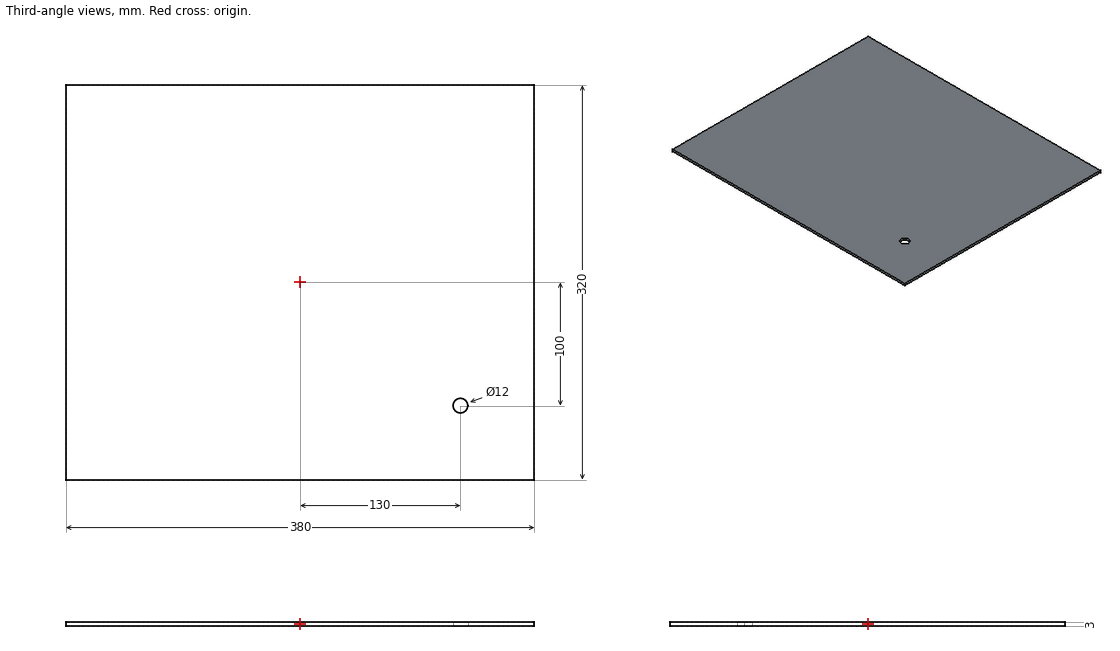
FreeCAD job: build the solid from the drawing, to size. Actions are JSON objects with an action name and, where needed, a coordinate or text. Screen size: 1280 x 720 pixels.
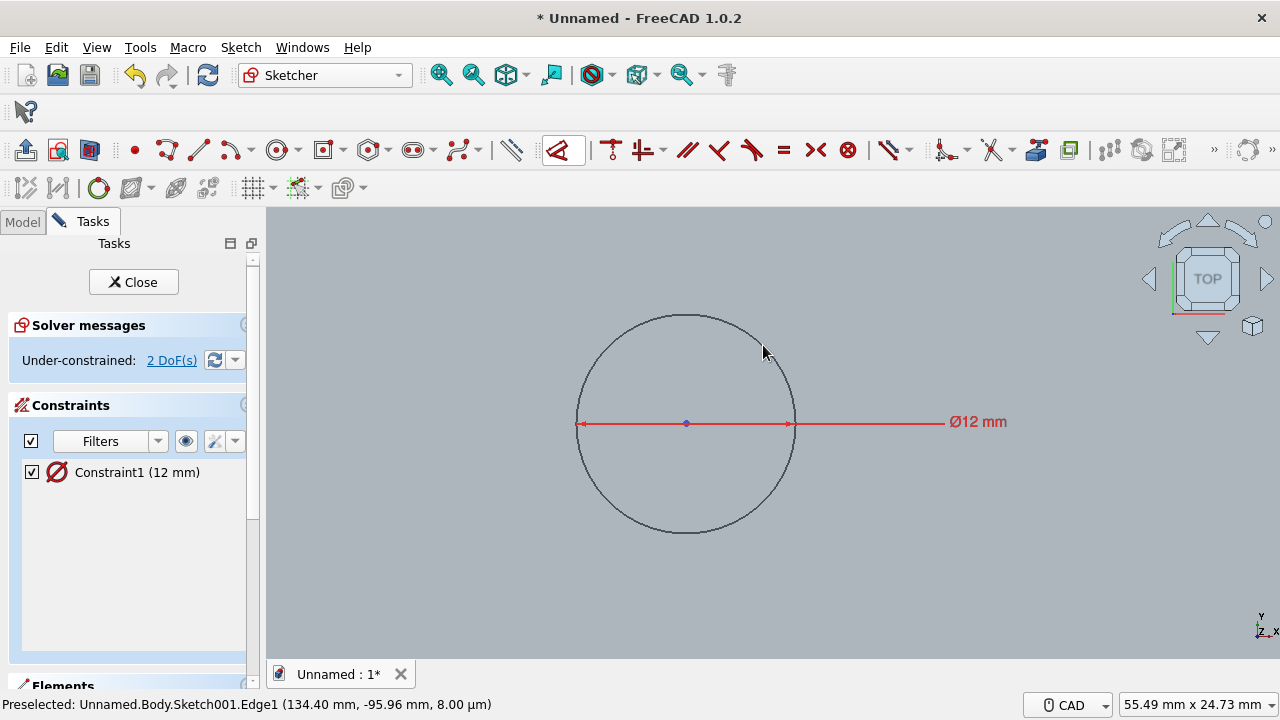
{"action": "left_click", "coordinate": [558, 150]}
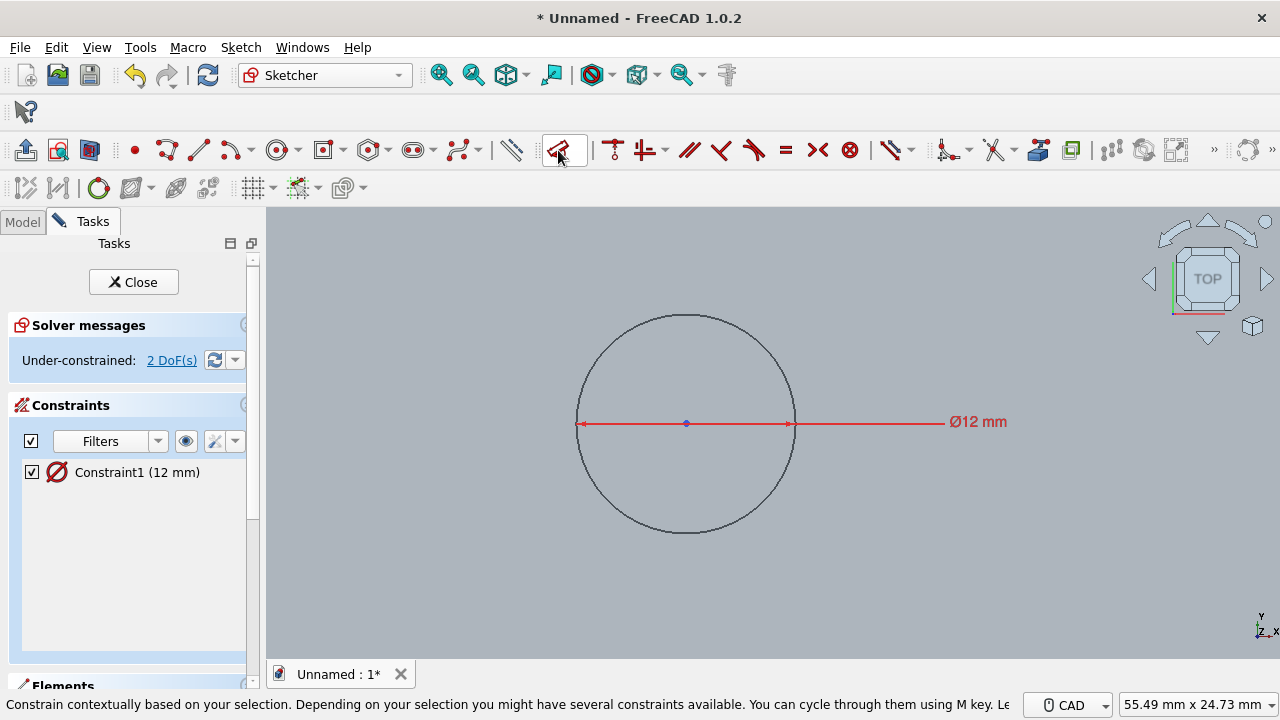
{"action": "left_click", "coordinate": [686, 424]}
{"action": "left_click", "coordinate": [490, 458]}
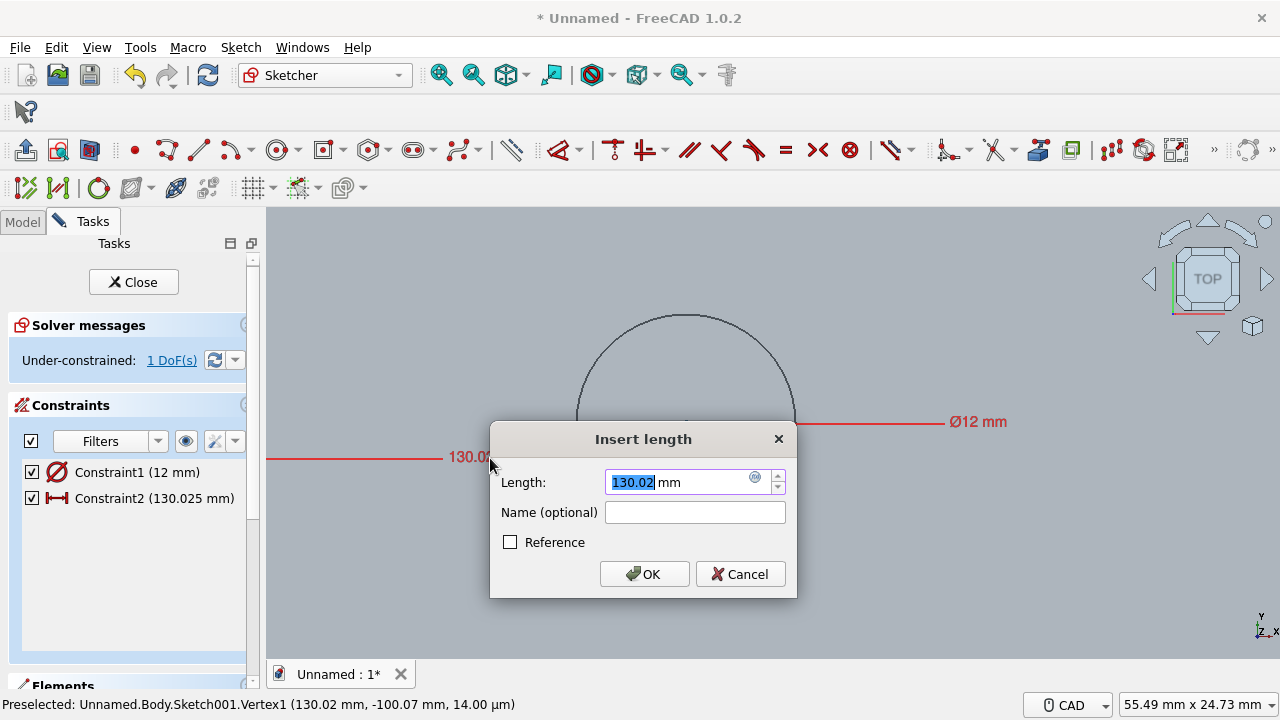
{"action": "type", "text": "130"}
{"action": "key", "text": "Return"}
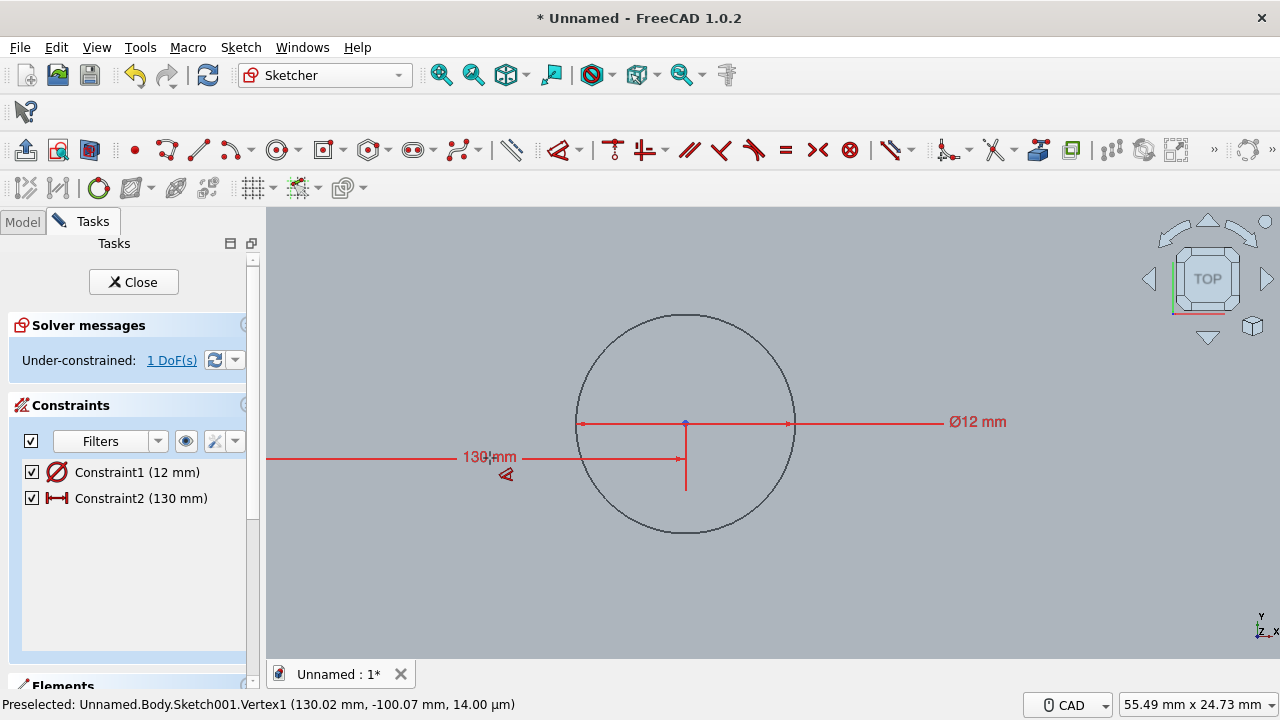
{"action": "left_click", "coordinate": [686, 424]}
{"action": "left_click", "coordinate": [720, 286]}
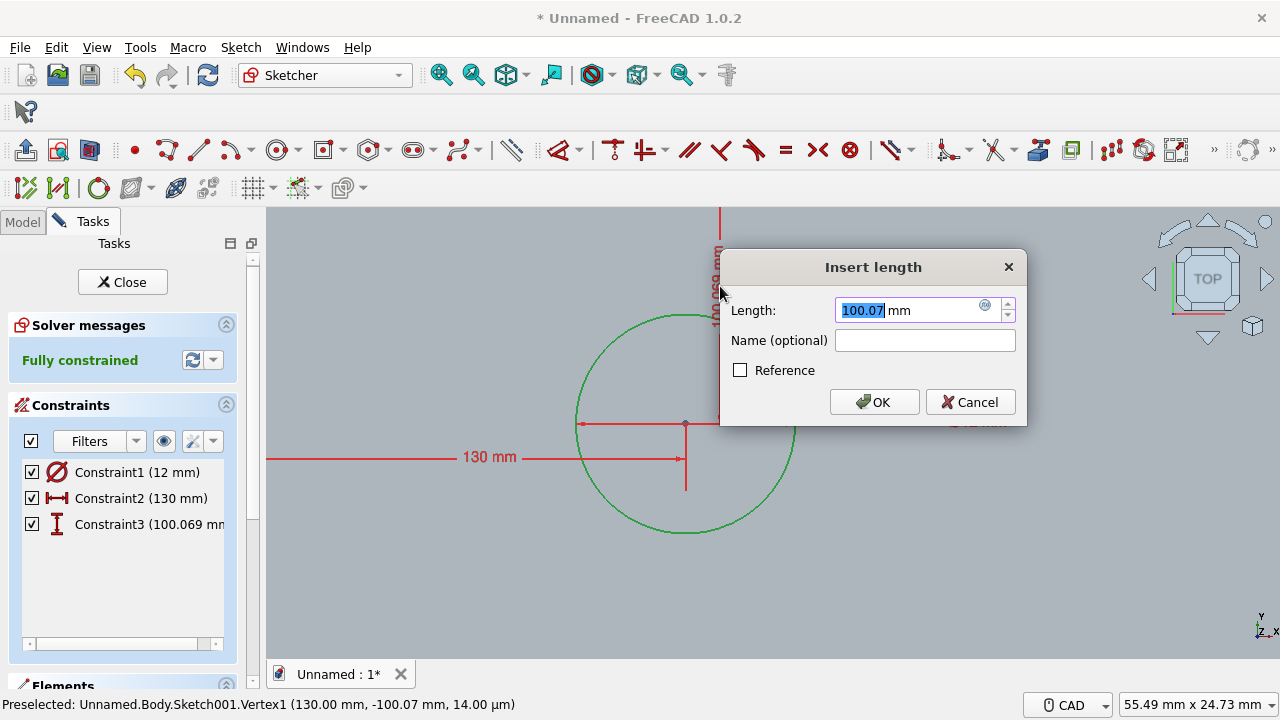
{"action": "type", "text": "100"}
{"action": "key", "text": "Return"}
{"action": "key", "text": "Escape"}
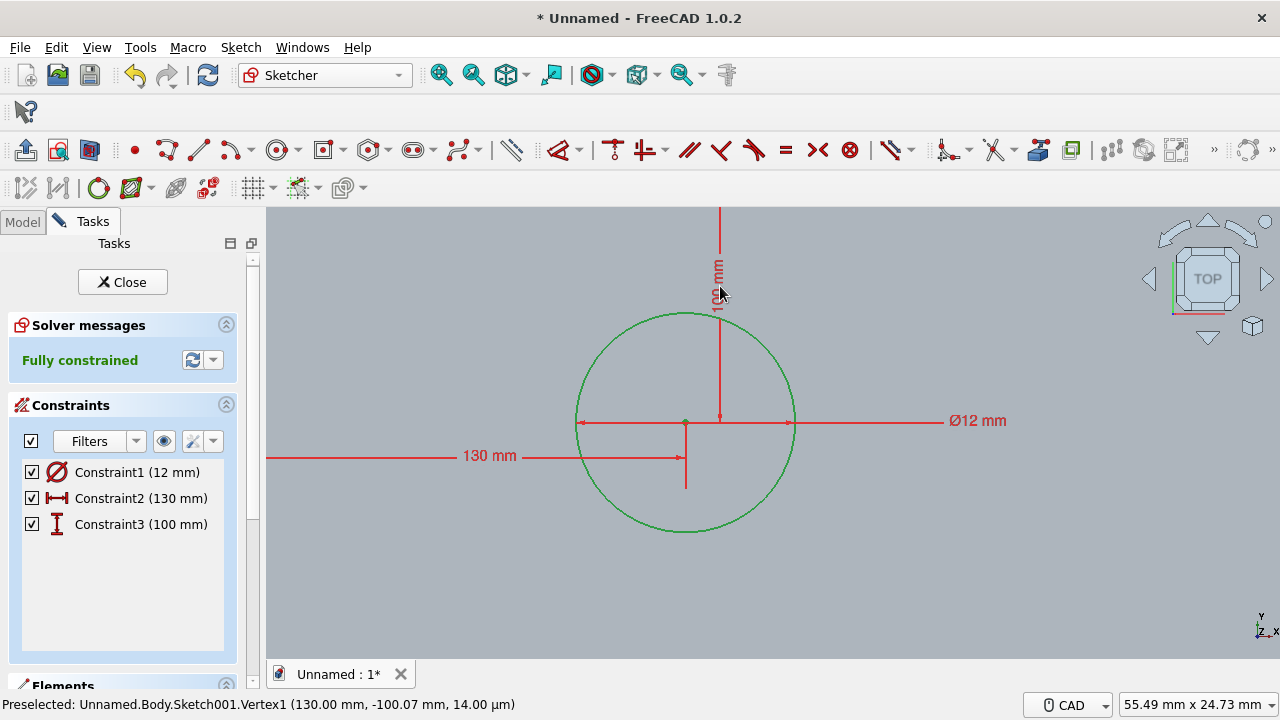
{"action": "left_click", "coordinate": [123, 282]}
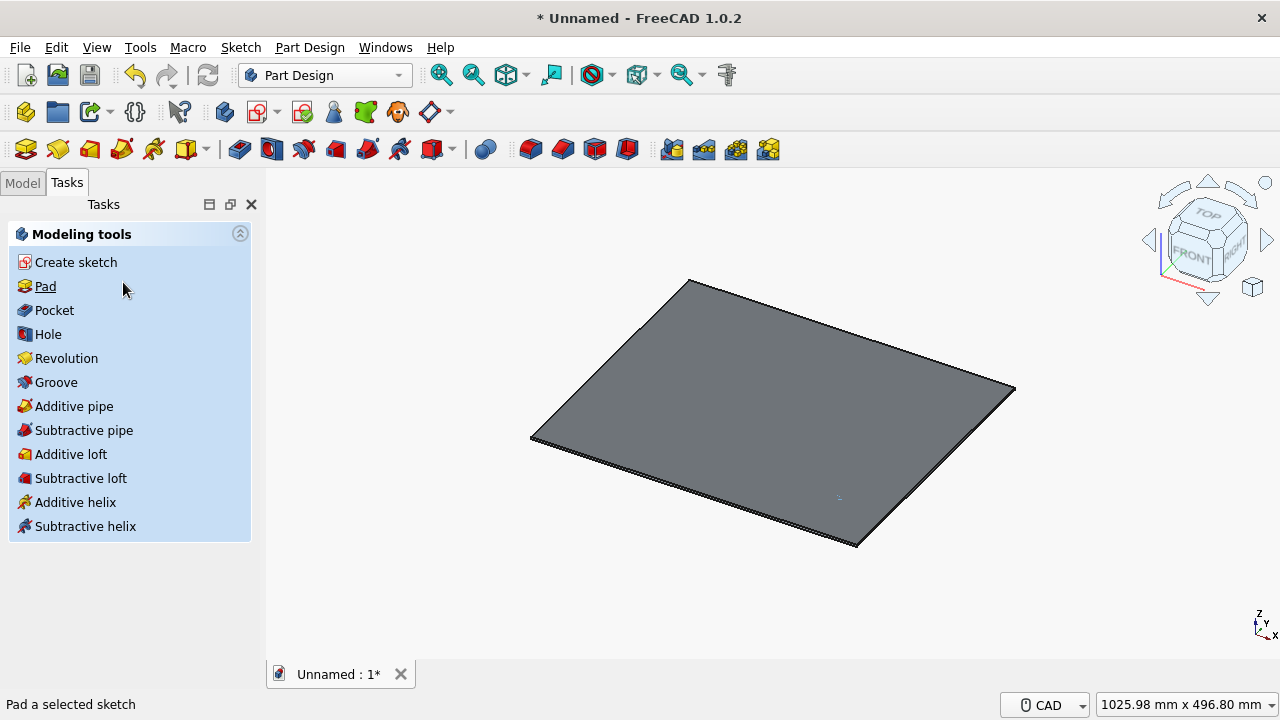
{"action": "left_click", "coordinate": [240, 150]}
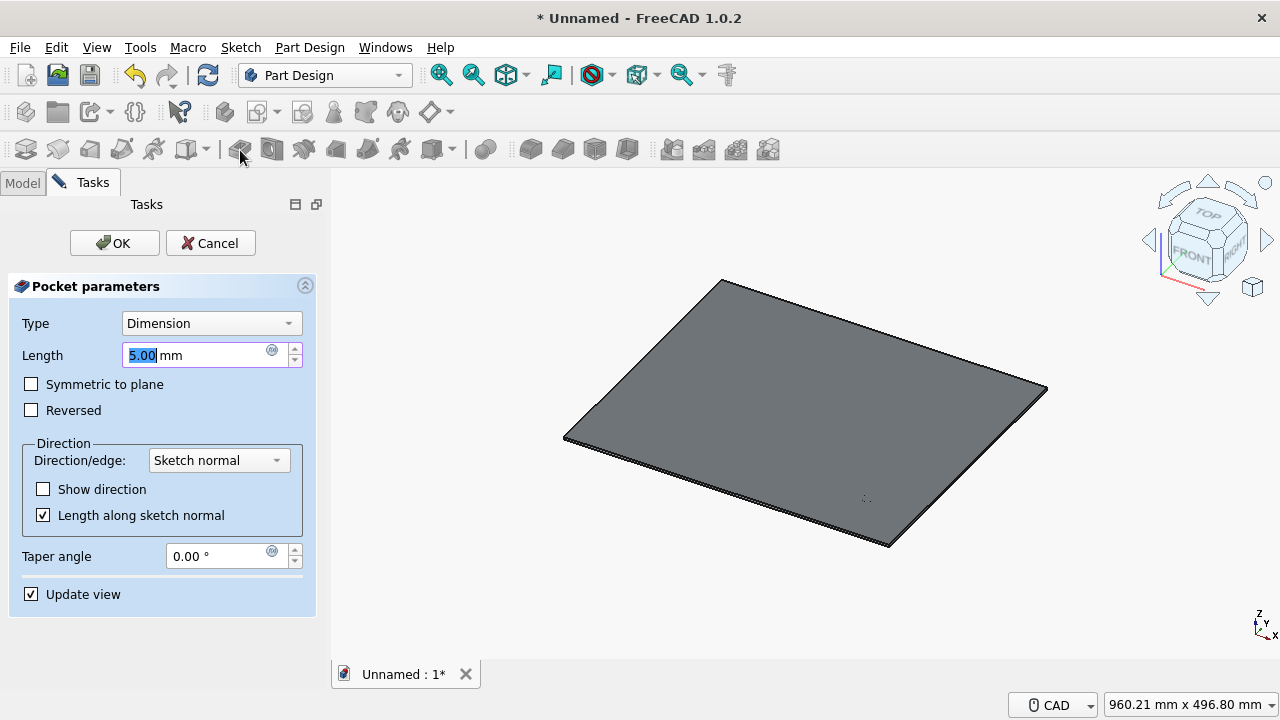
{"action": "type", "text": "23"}
{"action": "key", "text": "Tab"}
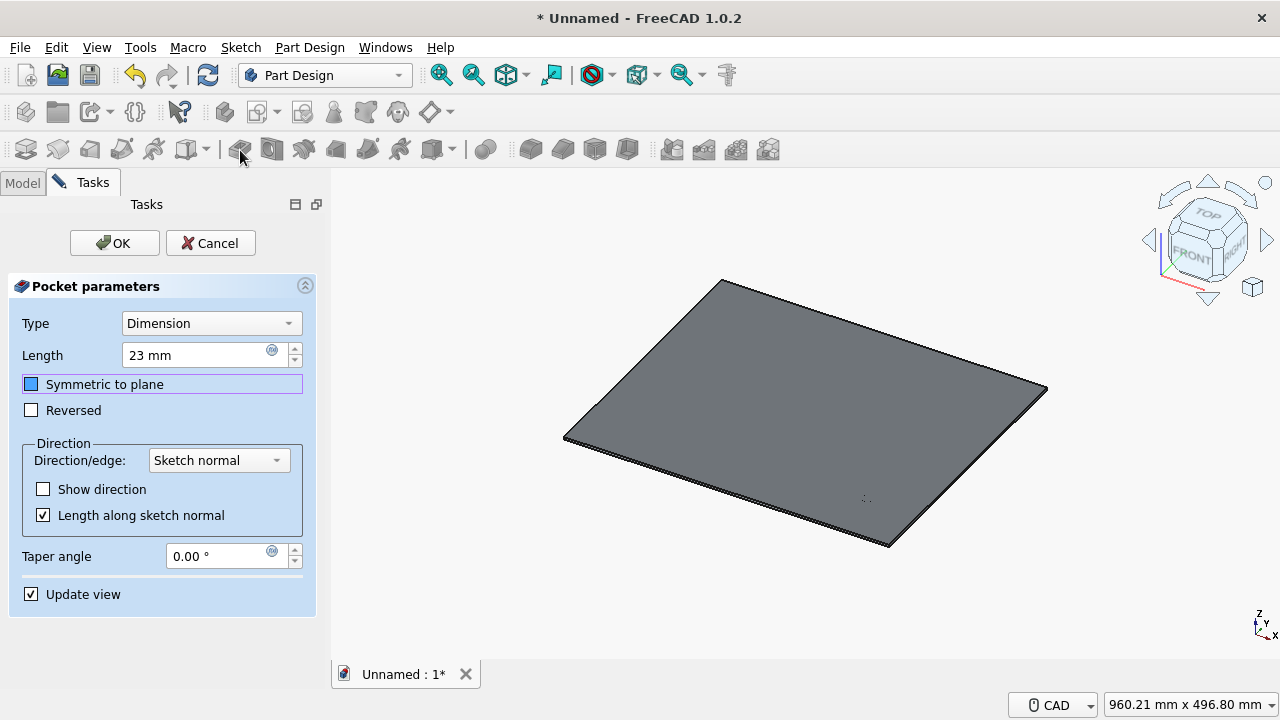
{"action": "left_click", "coordinate": [30, 384]}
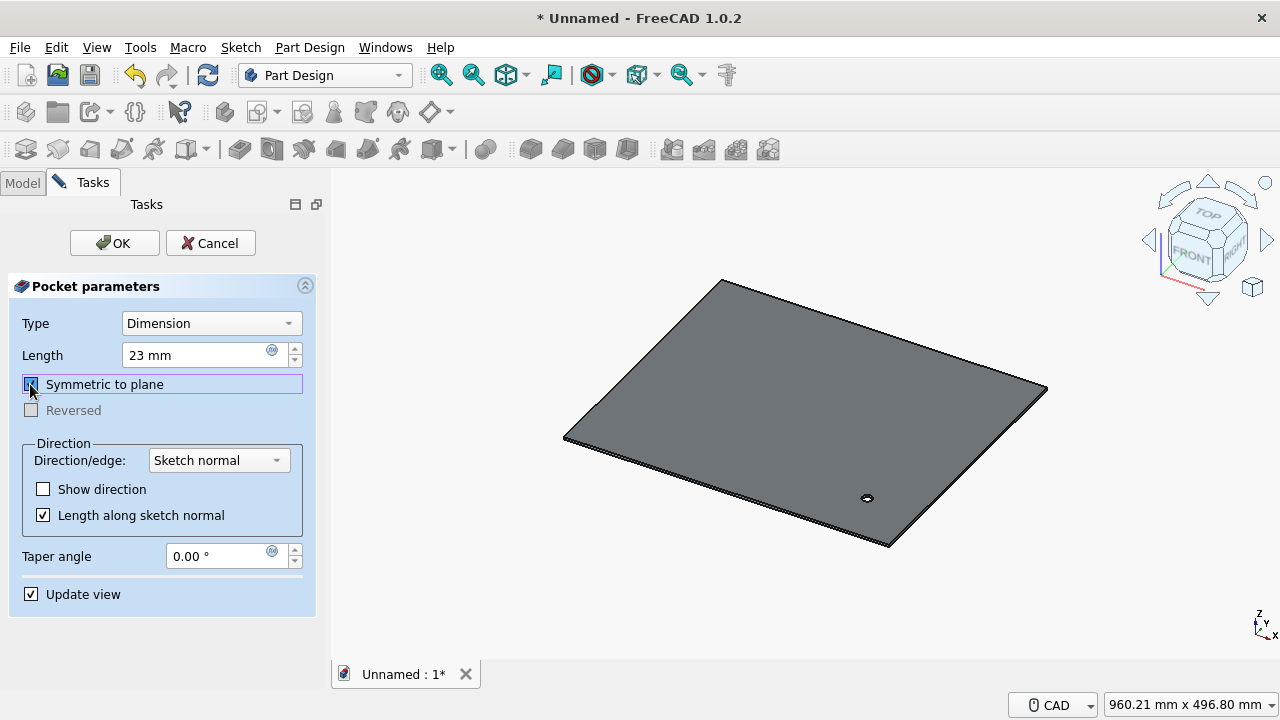
{"action": "left_click", "coordinate": [115, 243]}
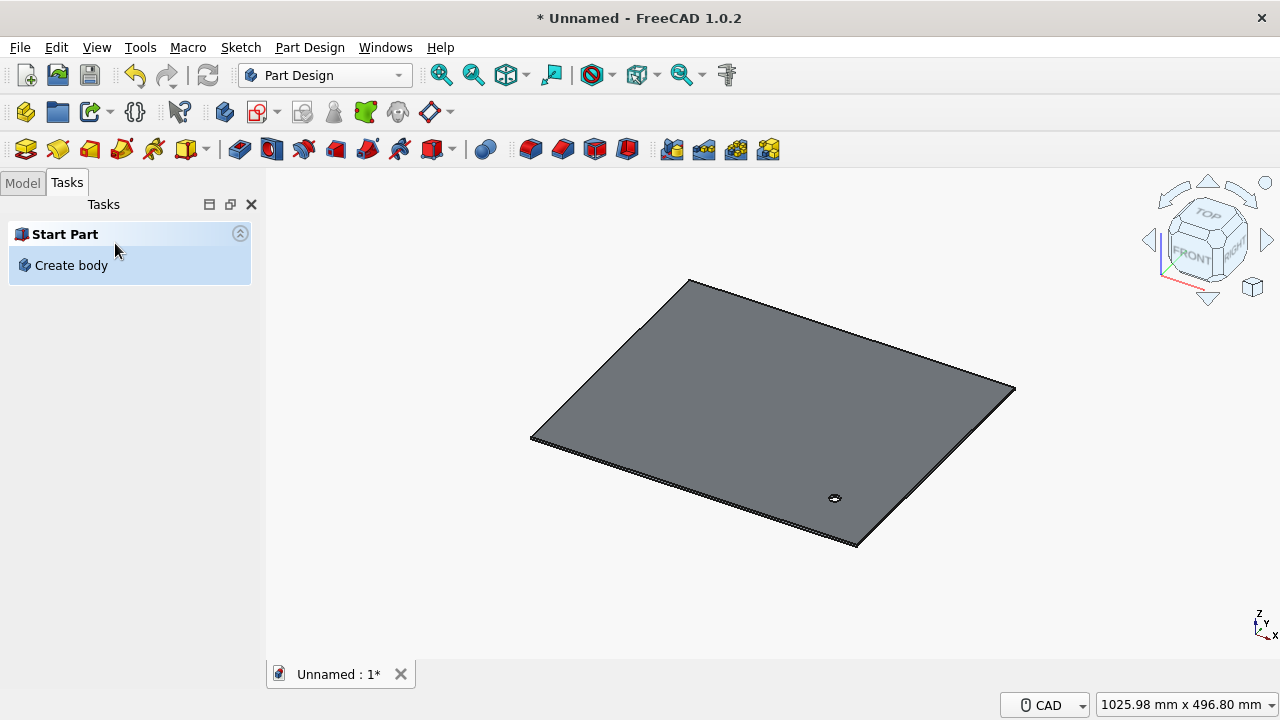
{"action": "key", "text": "0"}